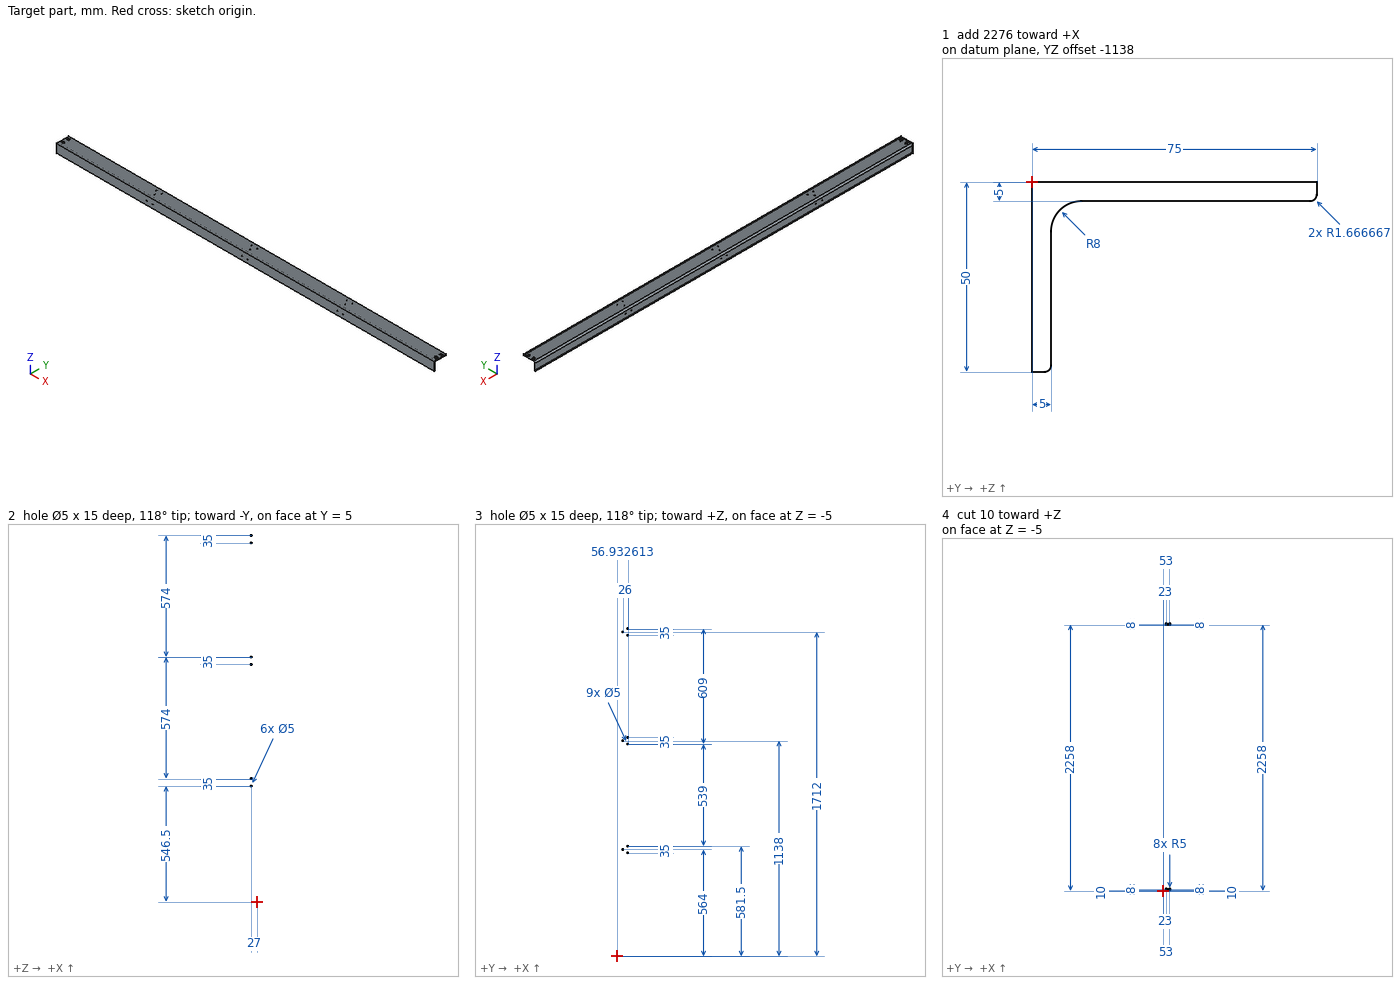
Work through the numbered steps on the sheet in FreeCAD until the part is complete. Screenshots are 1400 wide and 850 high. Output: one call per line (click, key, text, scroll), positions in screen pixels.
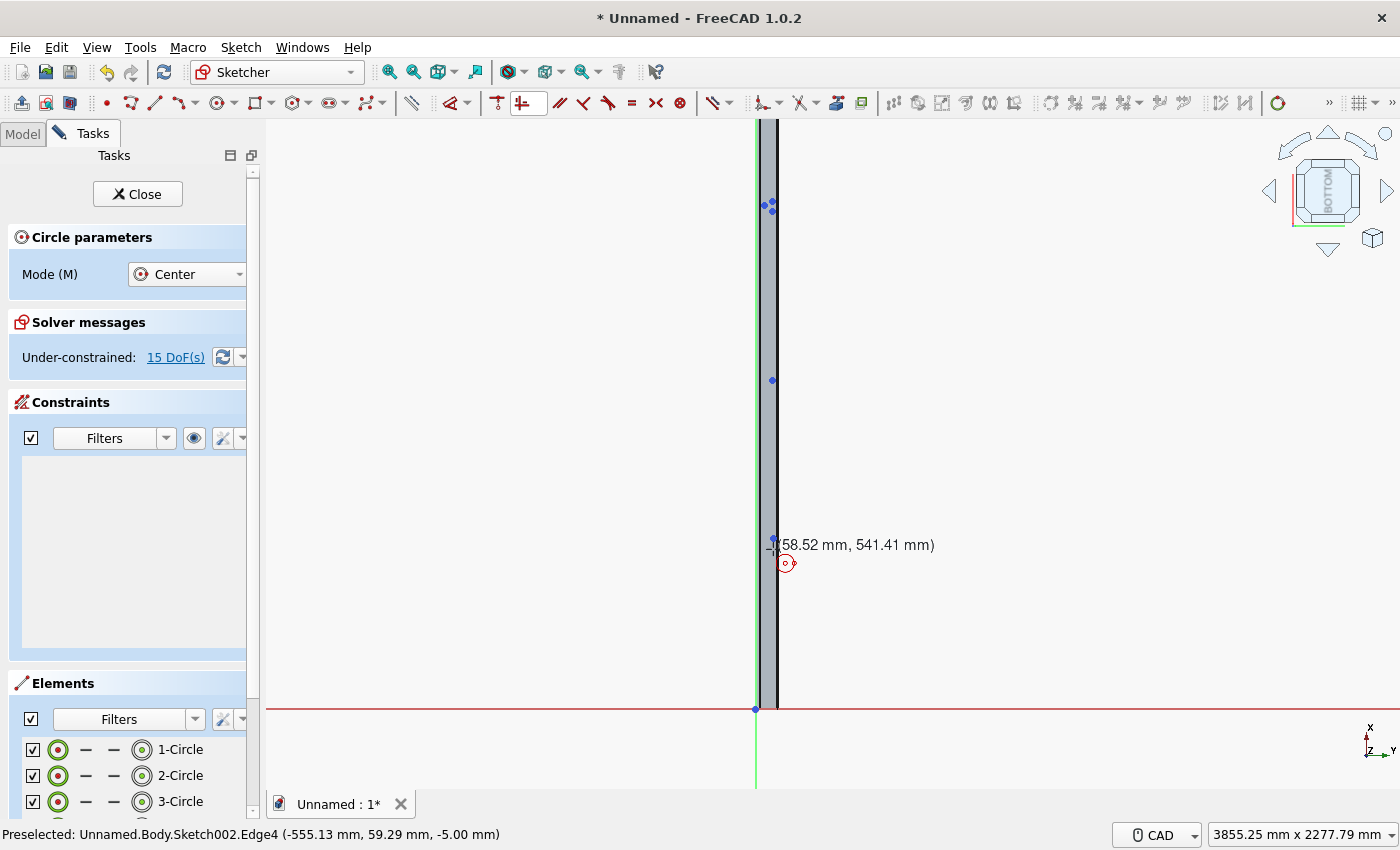
scroll(773, 549, up, 3)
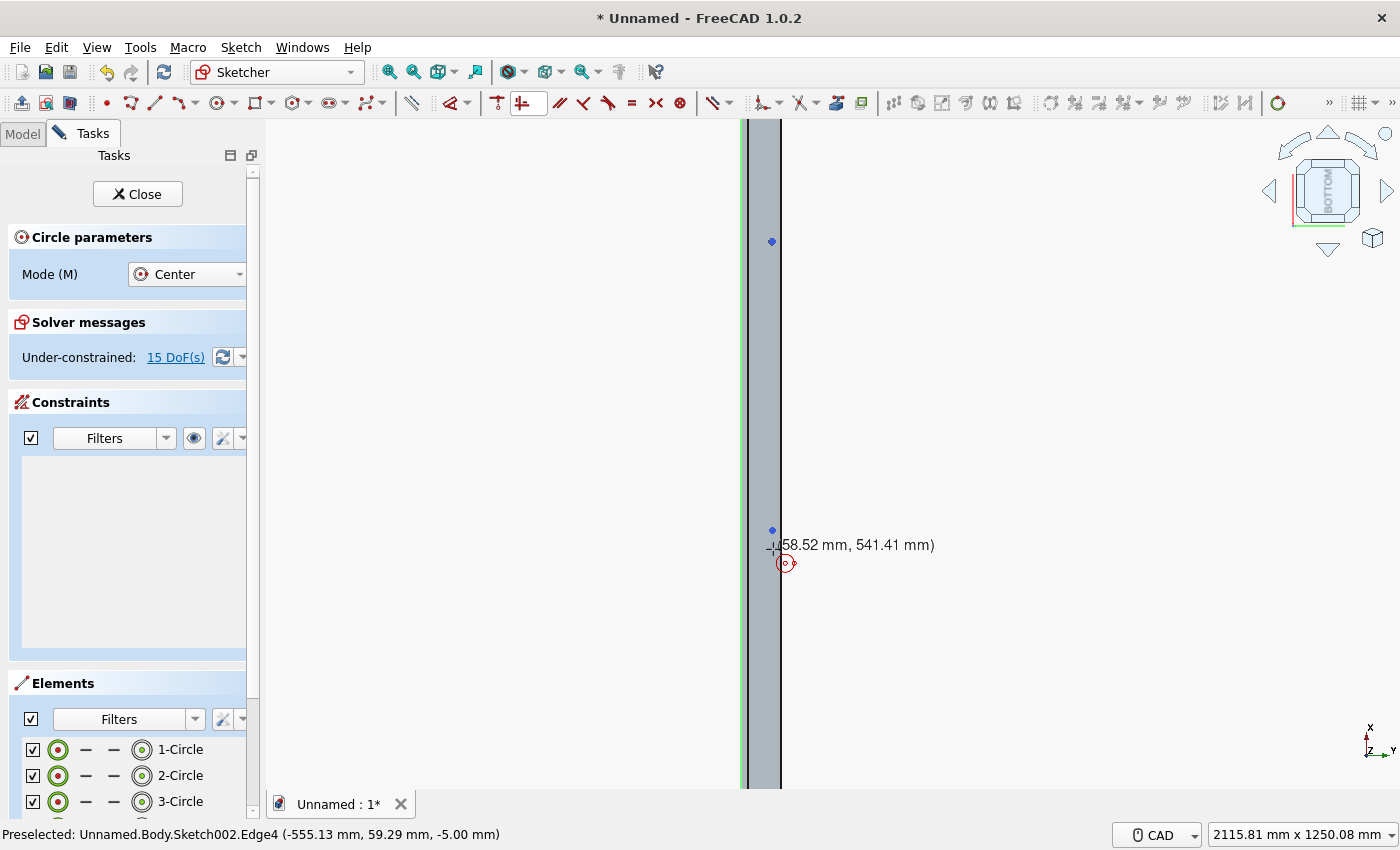
click(772, 548)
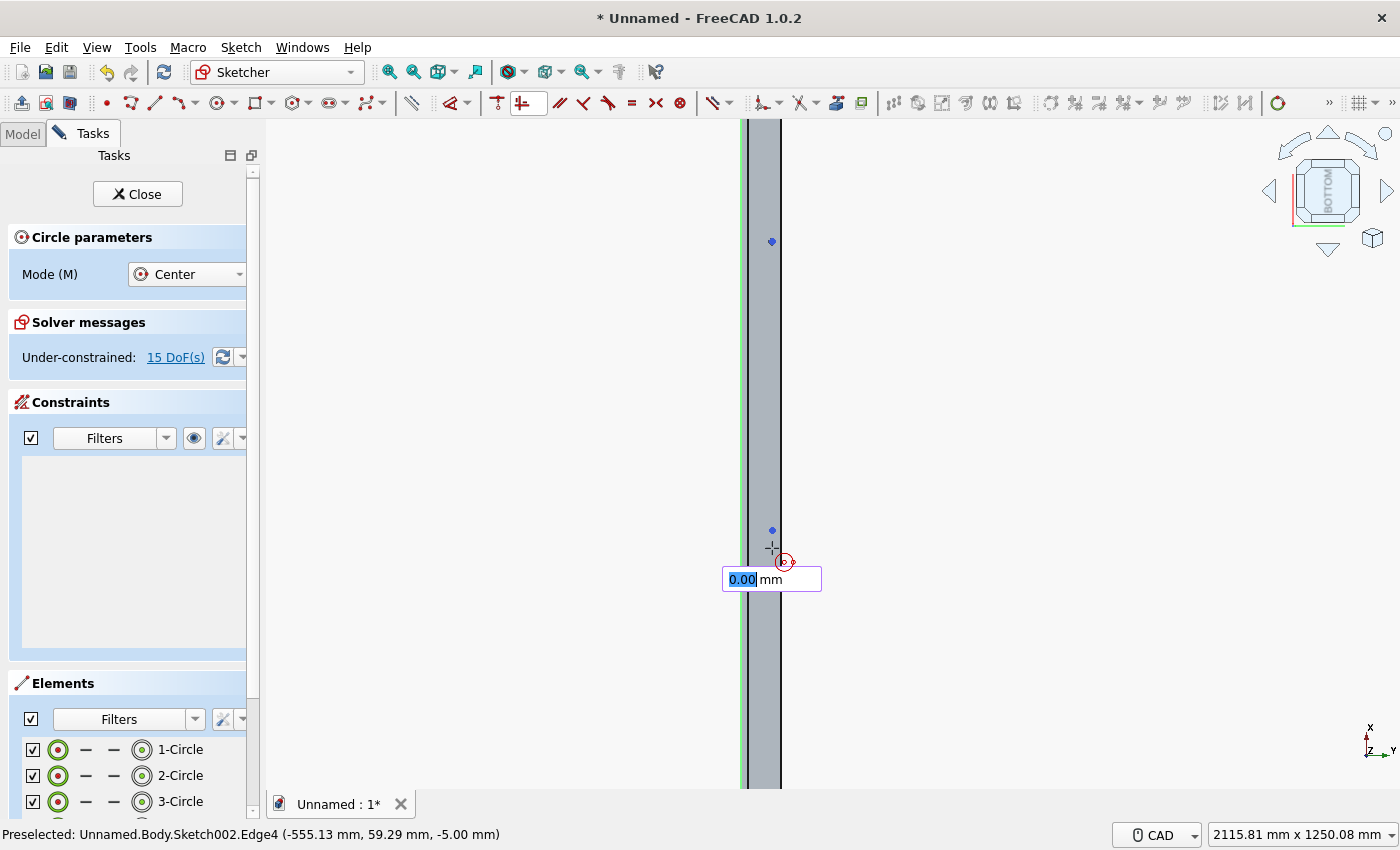
scroll(773, 547, up, 13)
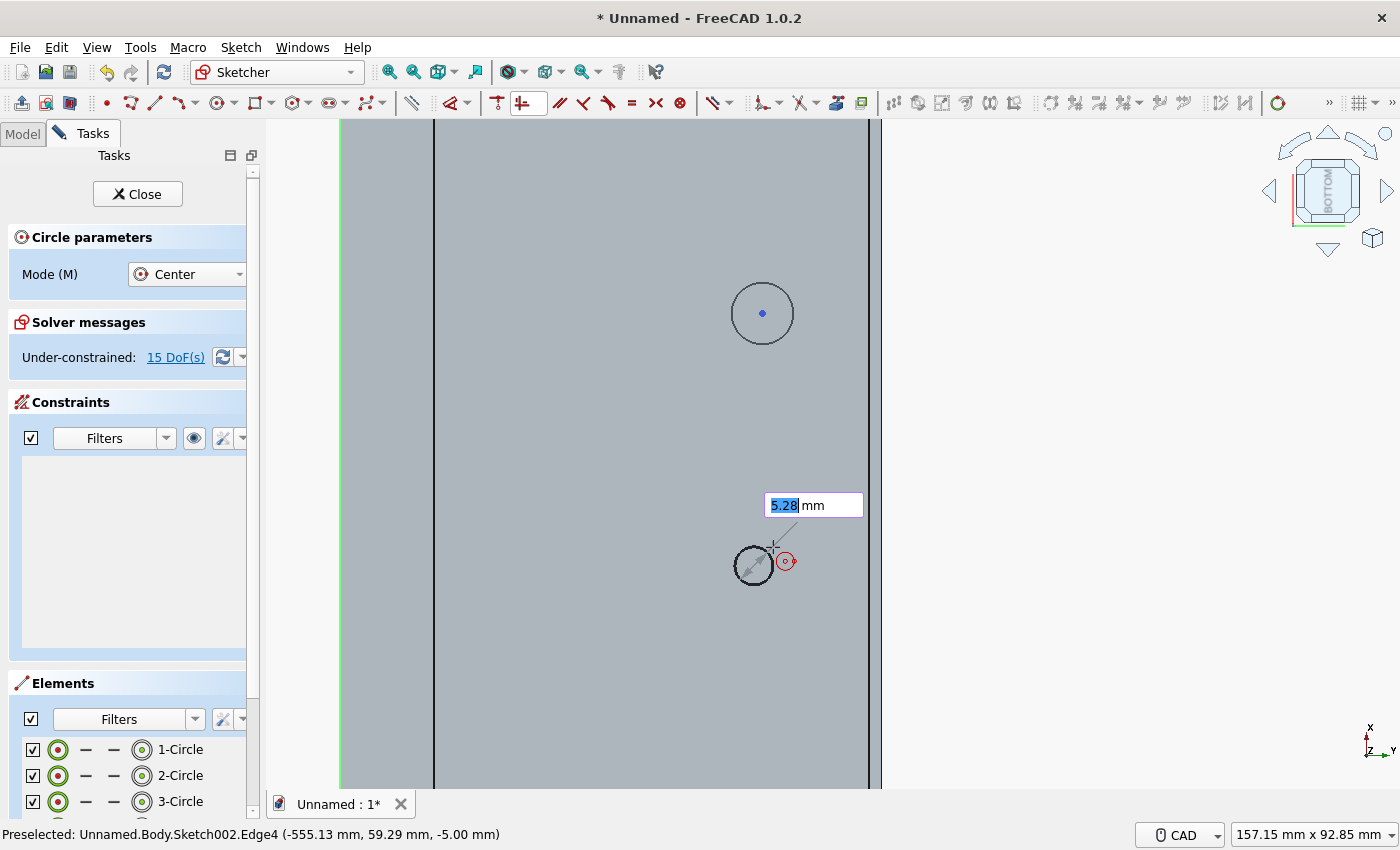
click(764, 534)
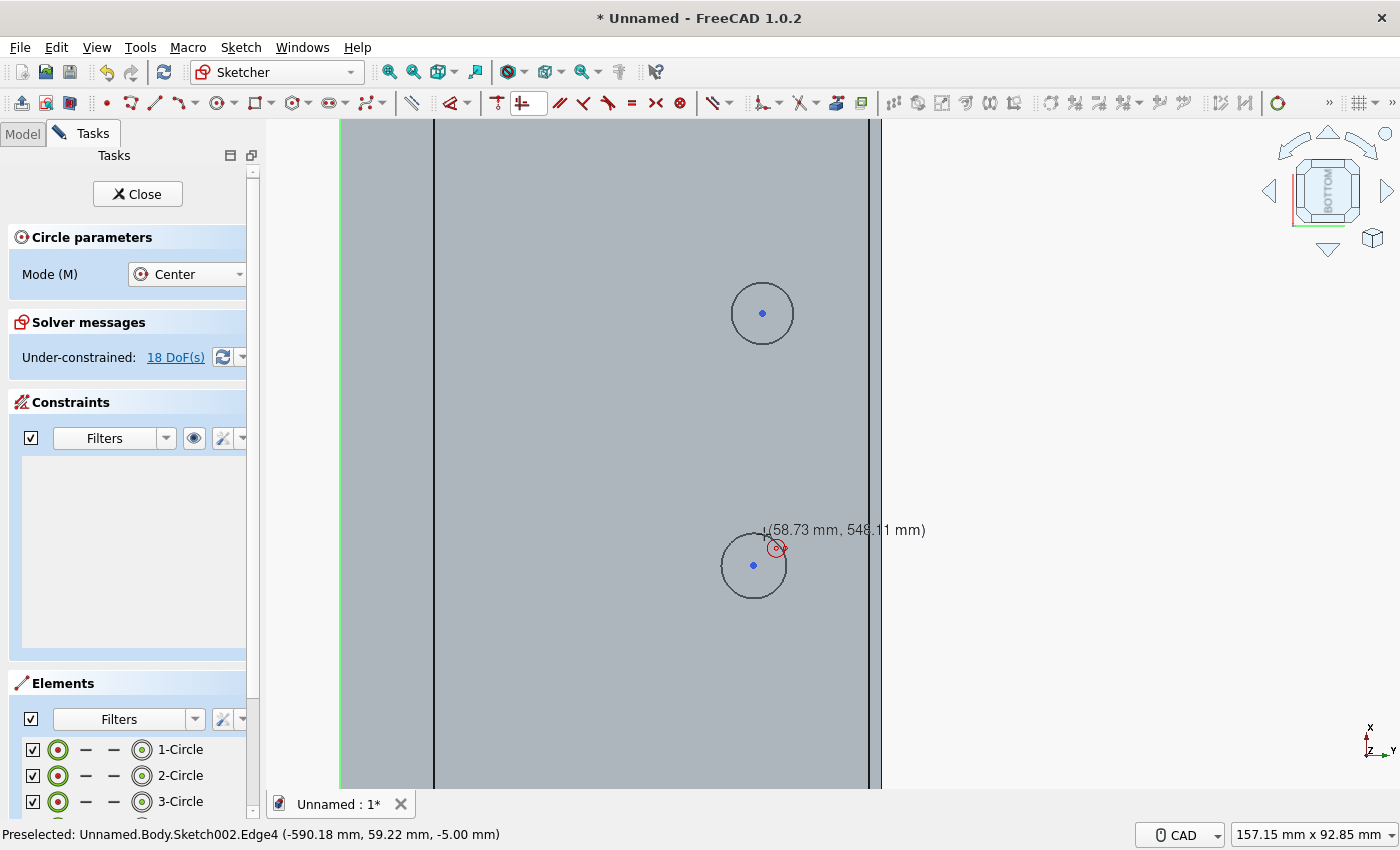
scroll(563, 420, up, 2)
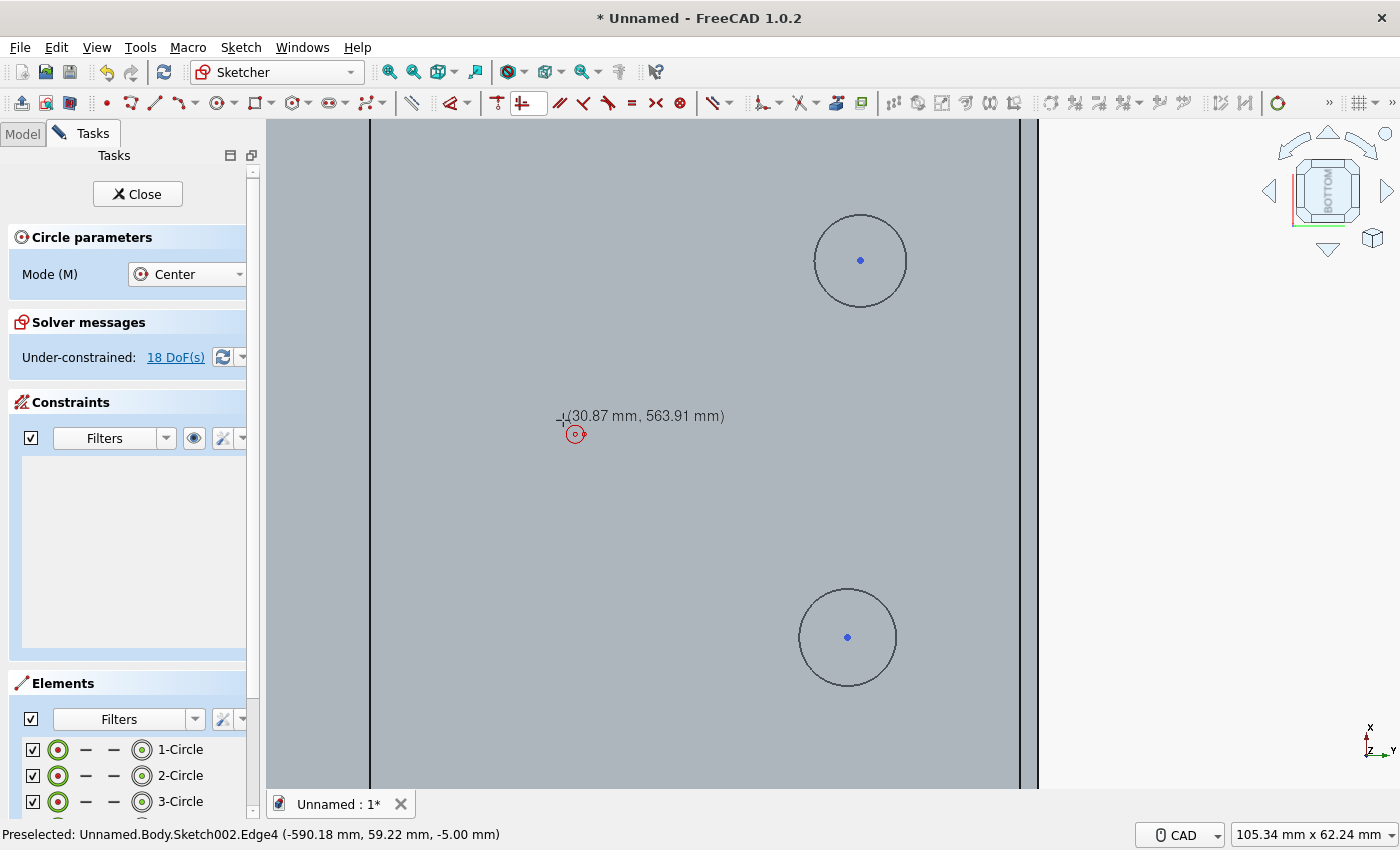
scroll(771, 546, down, 18)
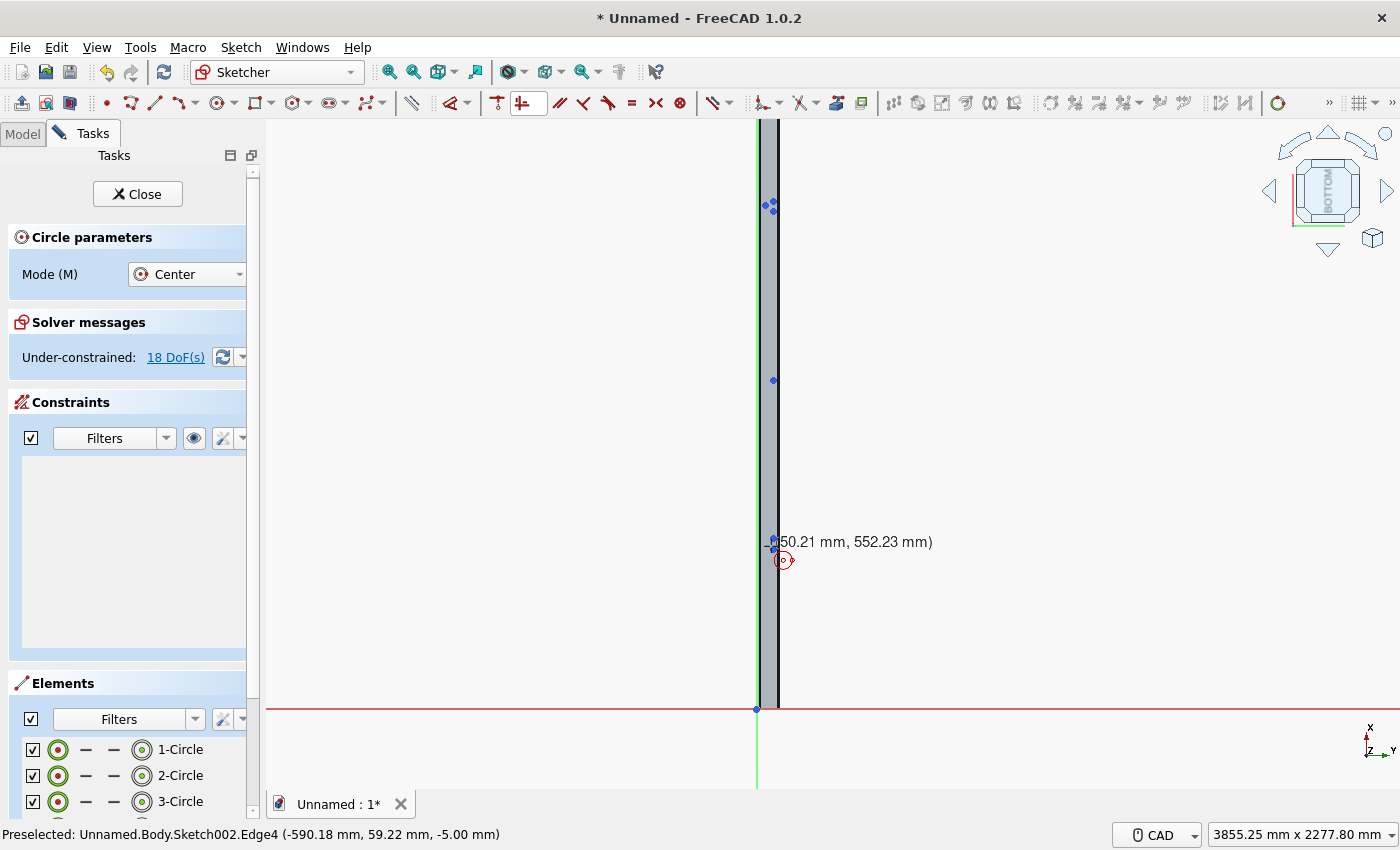
scroll(766, 543, up, 4)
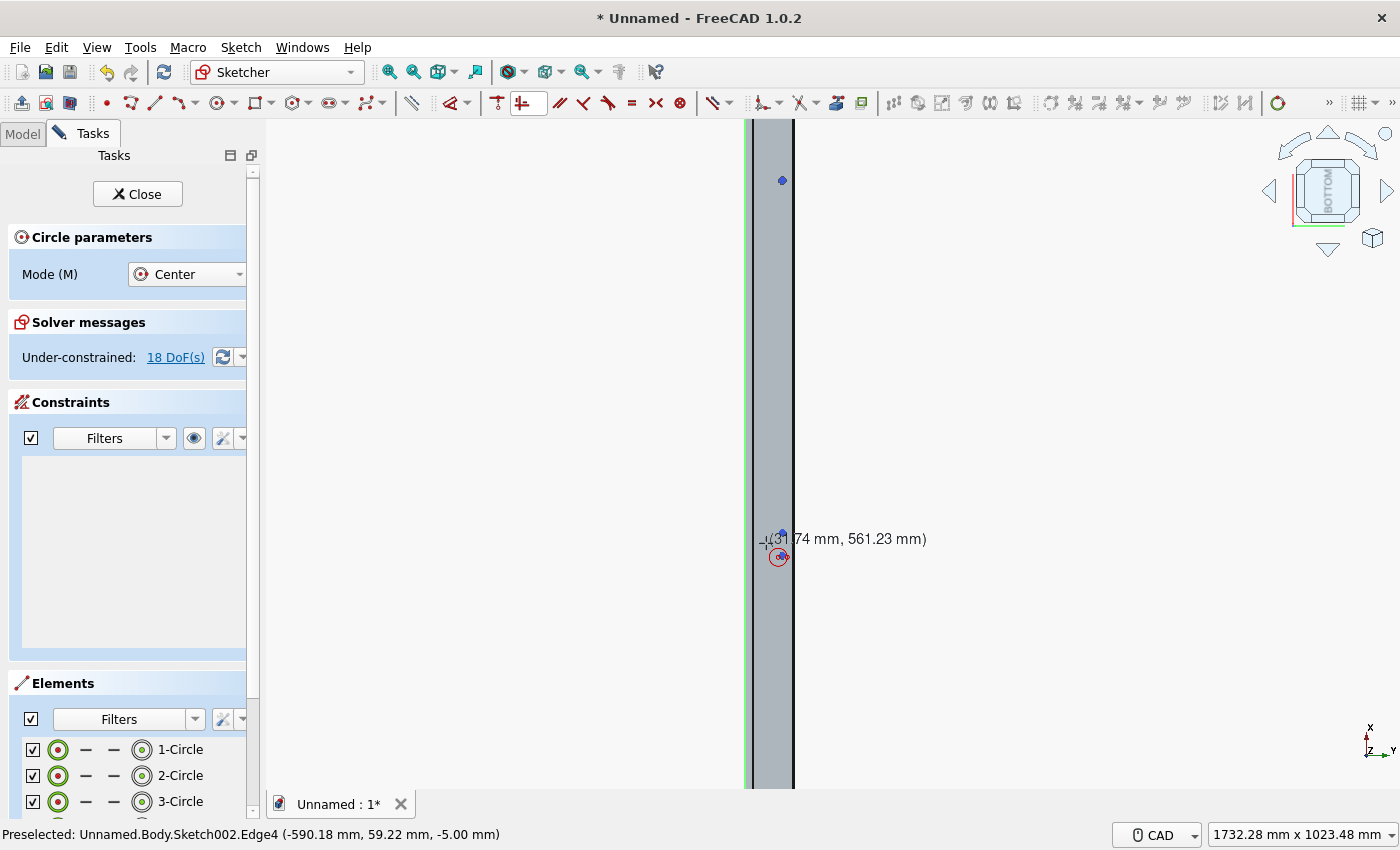
click(765, 543)